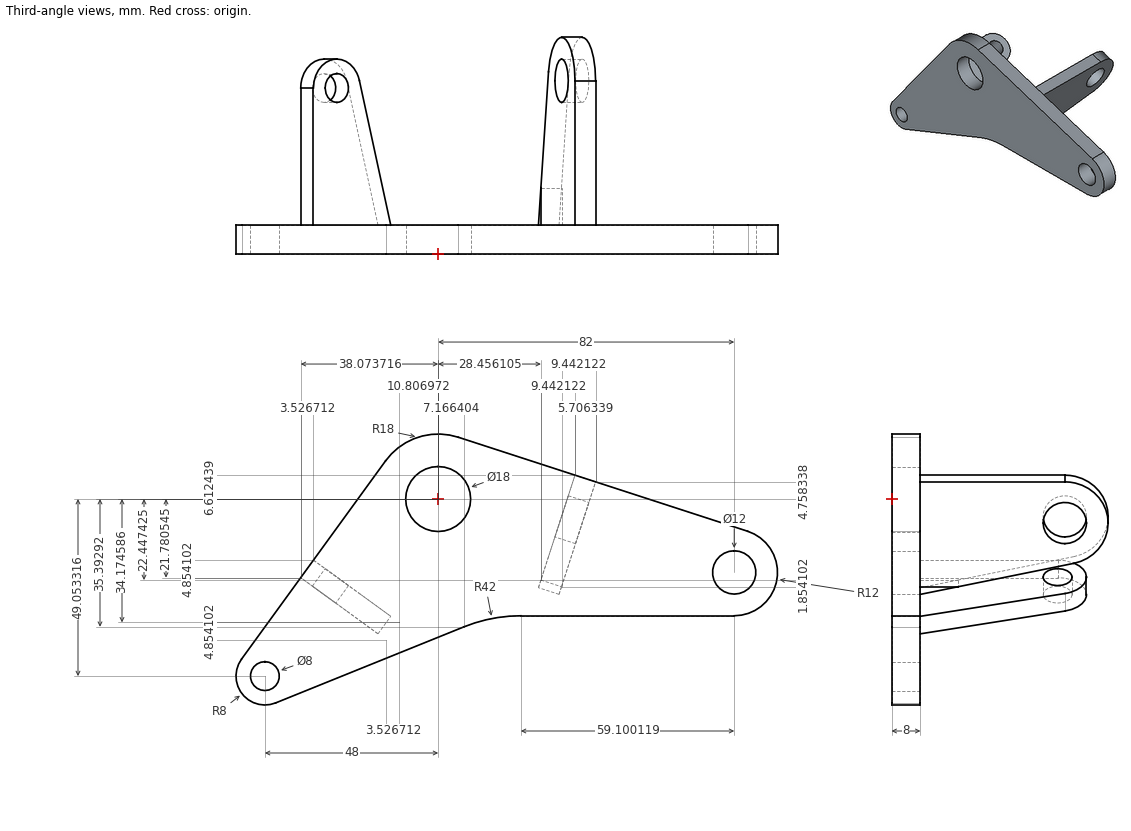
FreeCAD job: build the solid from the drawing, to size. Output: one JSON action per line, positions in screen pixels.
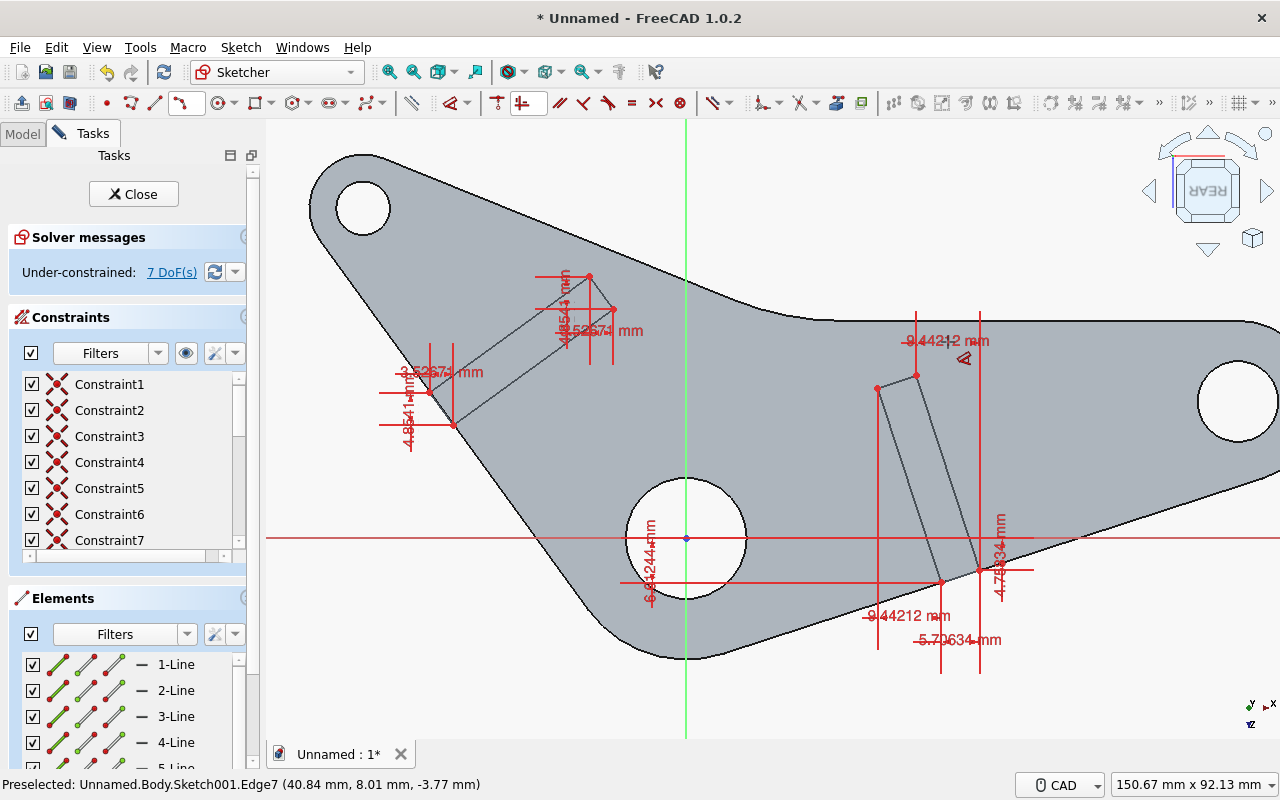
{"action": "scroll", "coordinate": [905, 380], "scroll_direction": "up", "scroll_amount": 6}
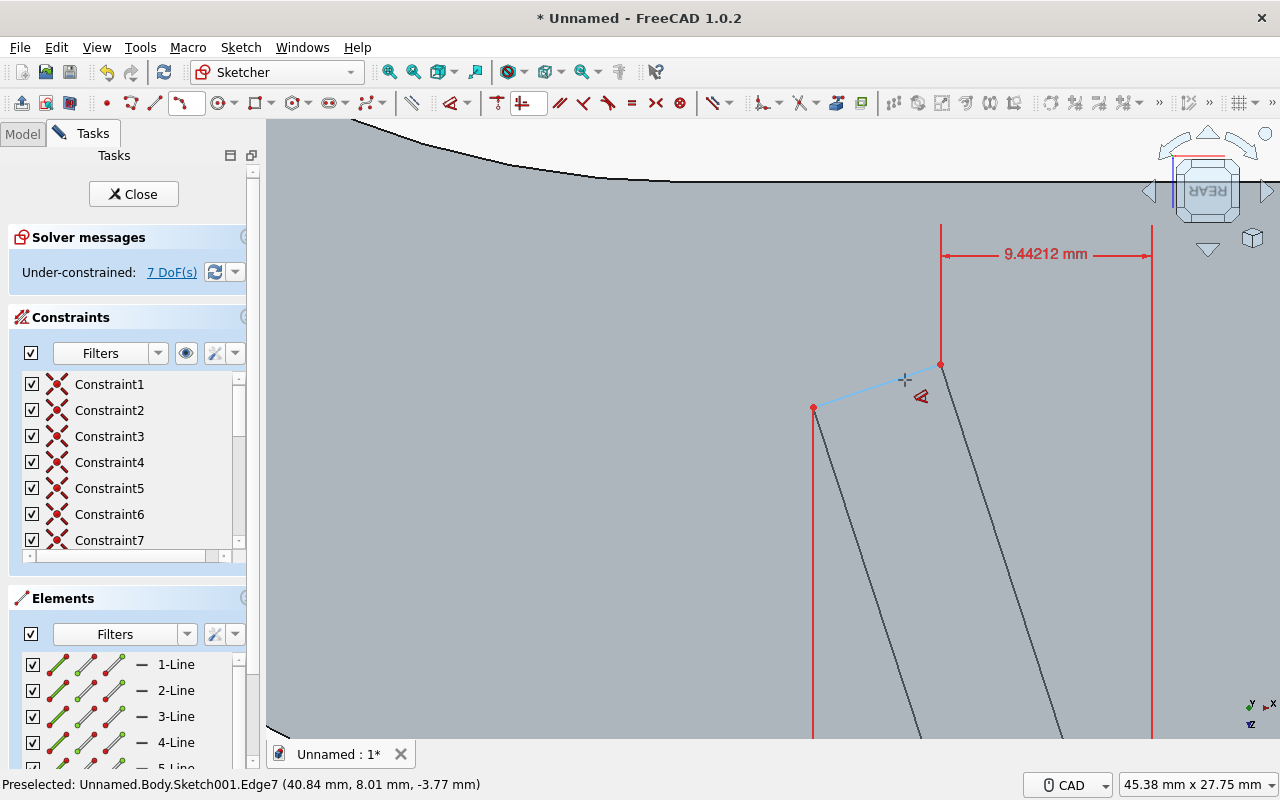
{"action": "left_click", "coordinate": [902, 378]}
{"action": "left_click", "coordinate": [975, 386]}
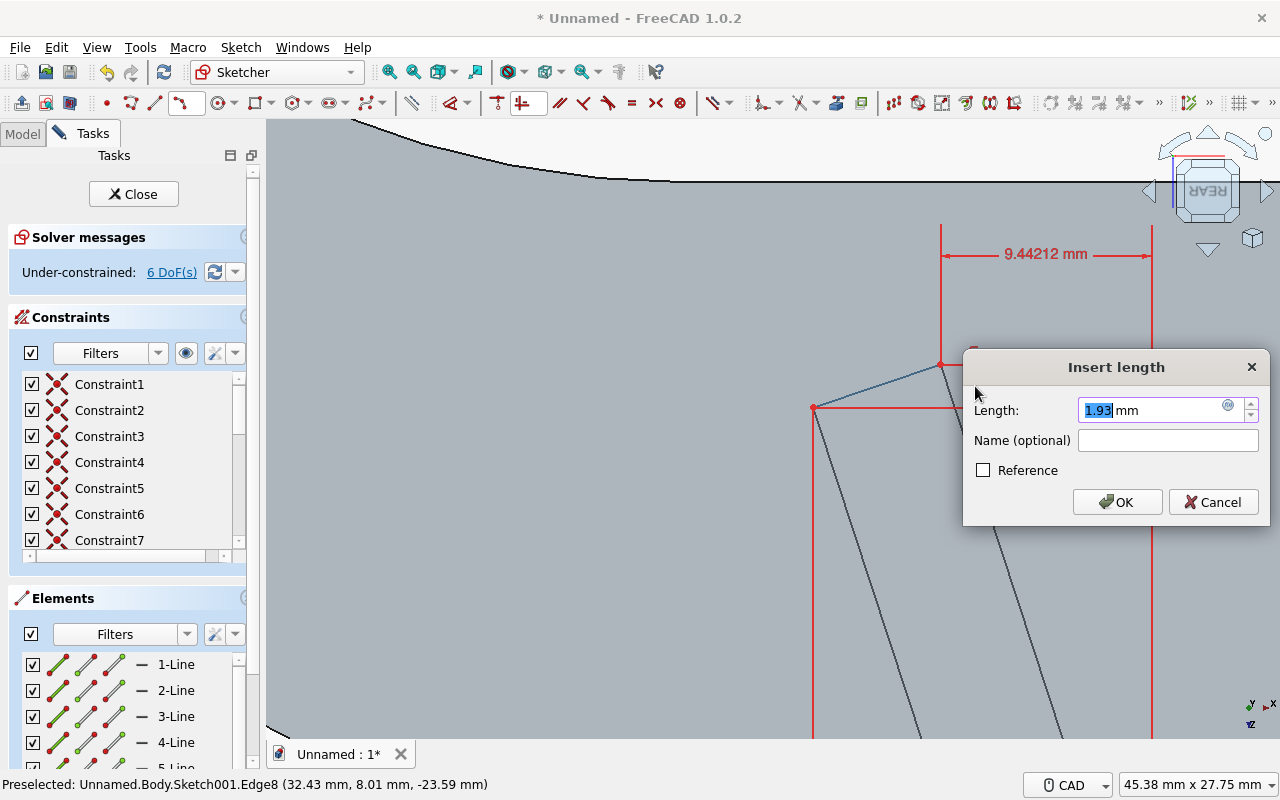
{"action": "type", "text": "1.854102"}
{"action": "key", "text": "Return"}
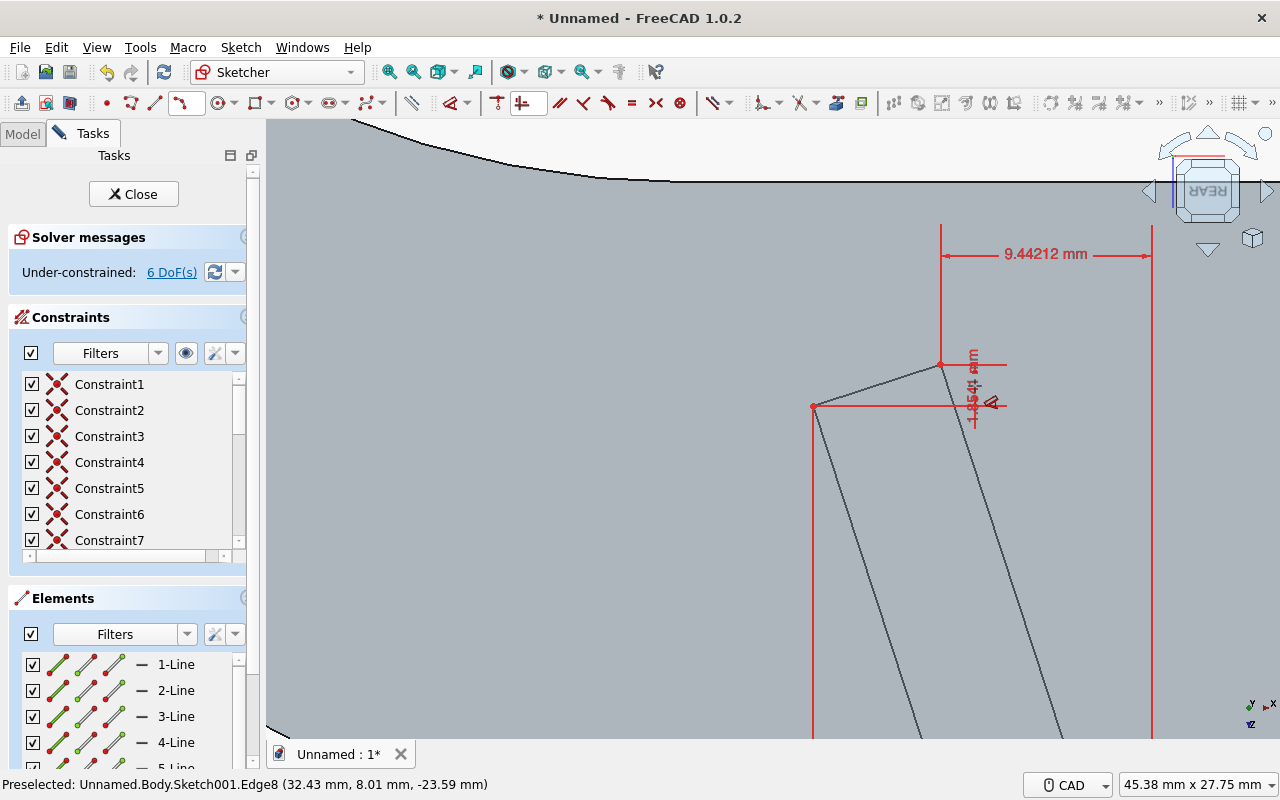
{"action": "scroll", "coordinate": [905, 380], "scroll_direction": "down", "scroll_amount": 6}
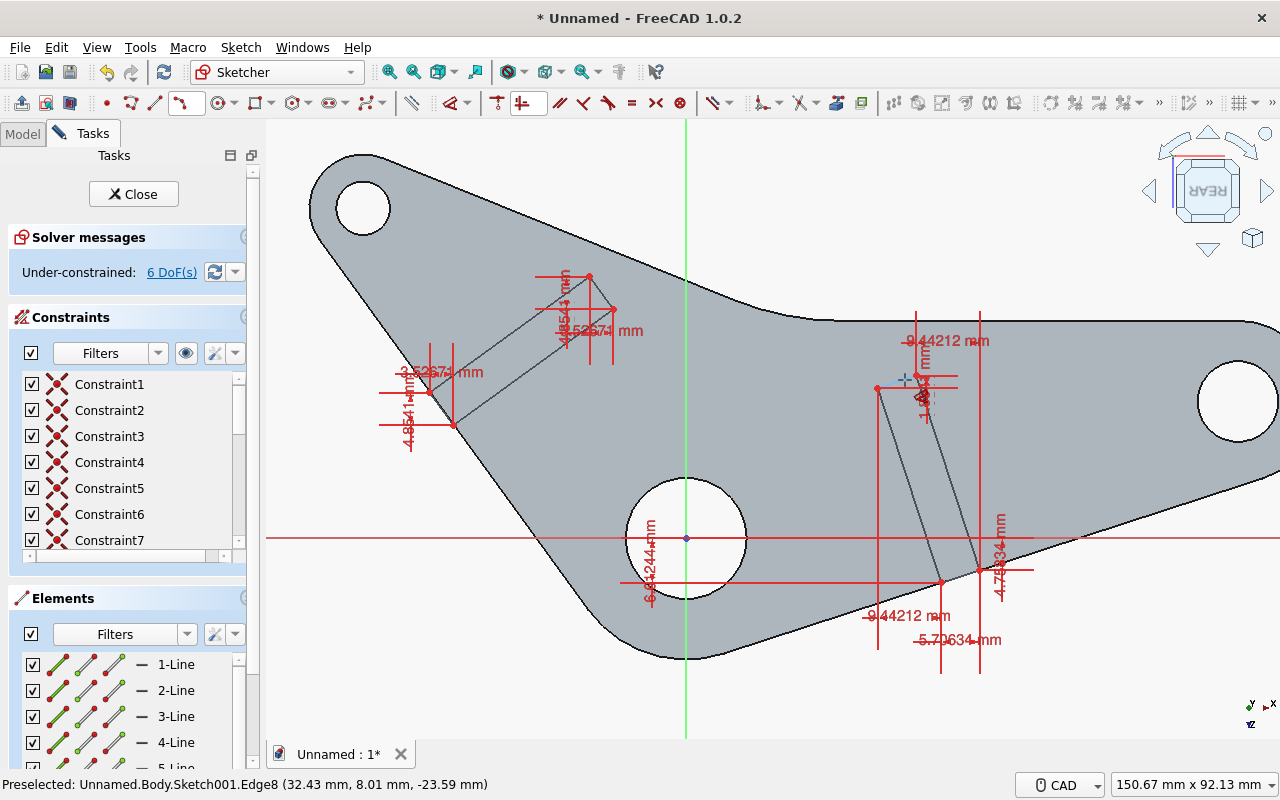
{"action": "left_click", "coordinate": [613, 309]}
{"action": "left_click", "coordinate": [650, 275]}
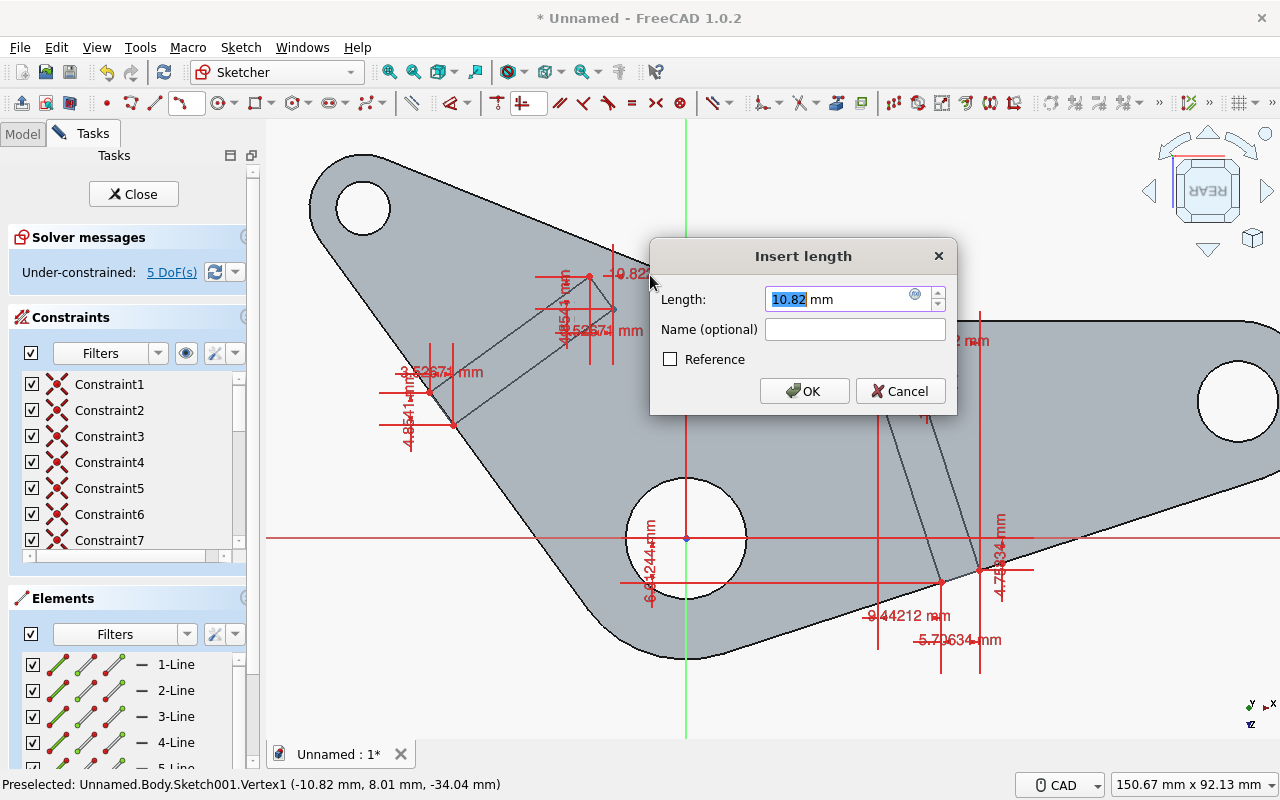
{"action": "type", "text": "10.806972"}
{"action": "key", "text": "Return"}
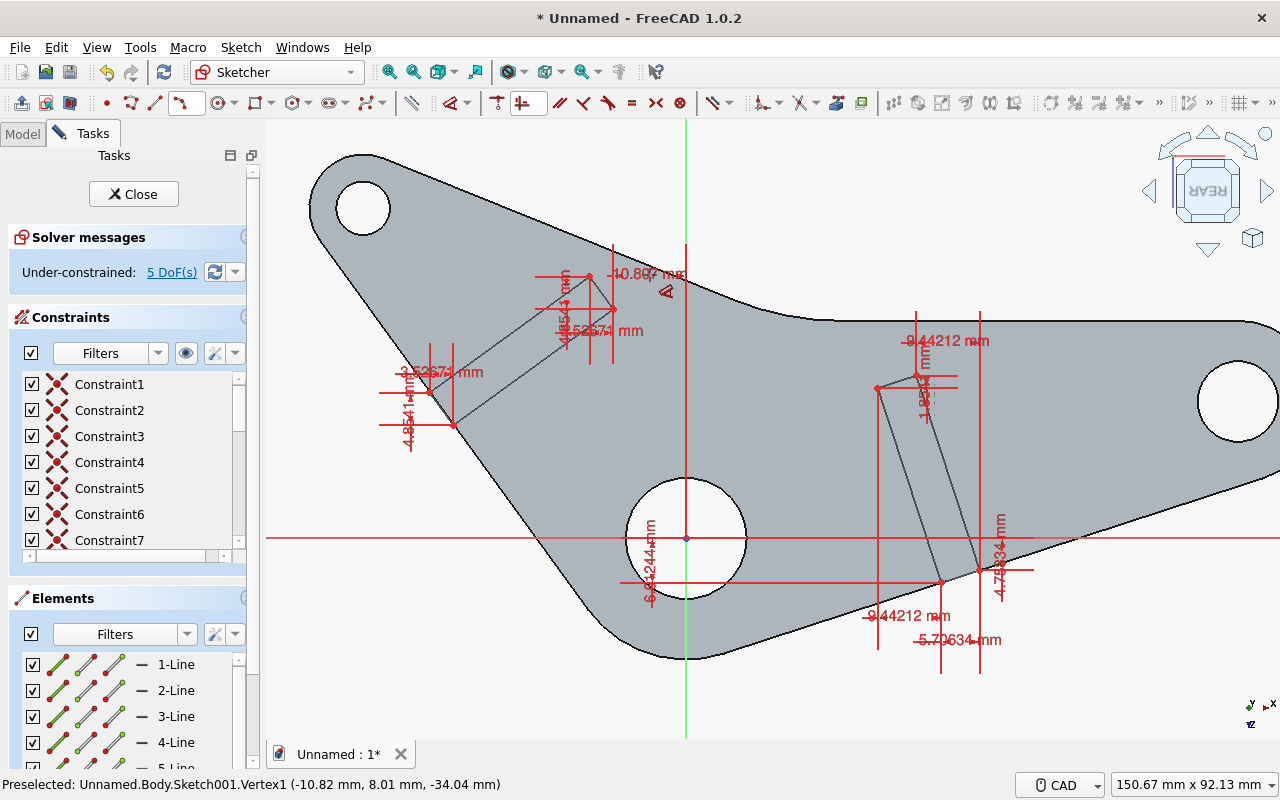
{"action": "left_click", "coordinate": [613, 309]}
{"action": "left_click", "coordinate": [579, 424]}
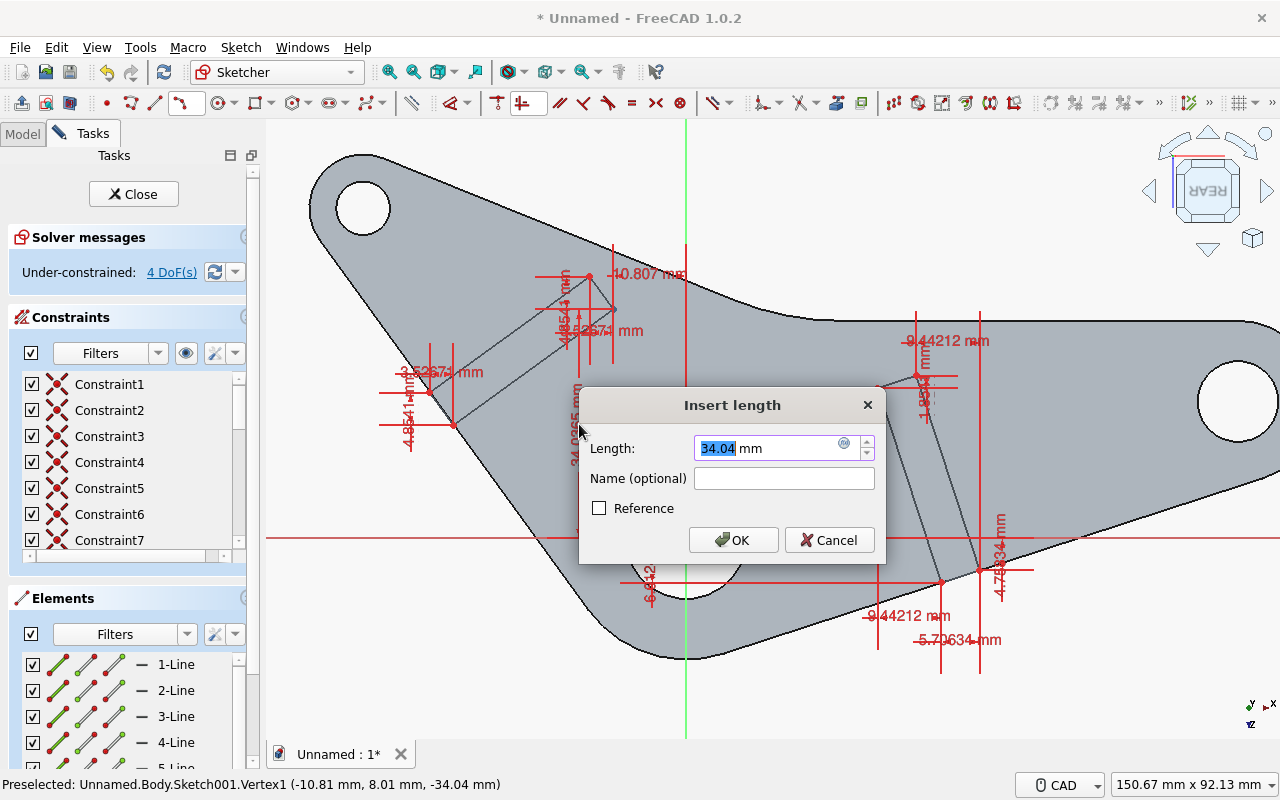
{"action": "type", "text": "34.174586"}
{"action": "key", "text": "Return"}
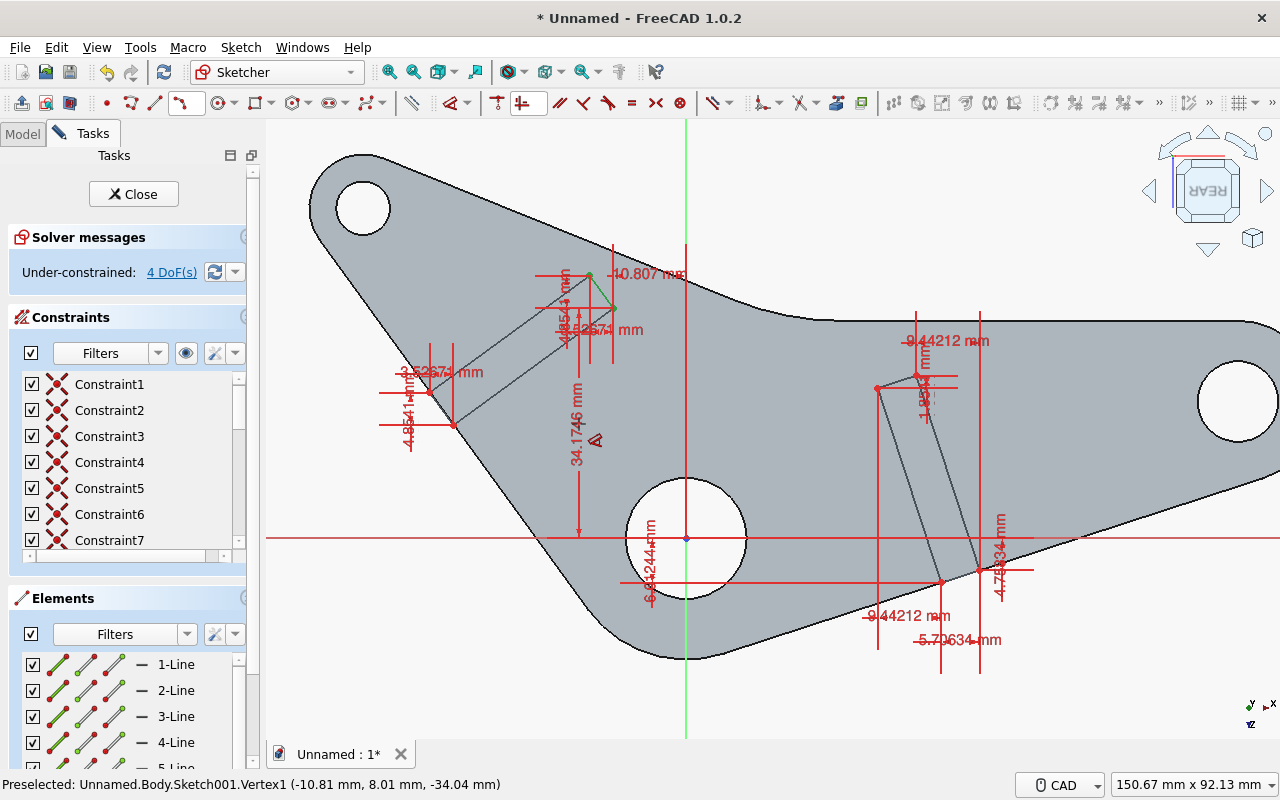
{"action": "left_click", "coordinate": [430, 393]}
{"action": "left_click", "coordinate": [558, 572]}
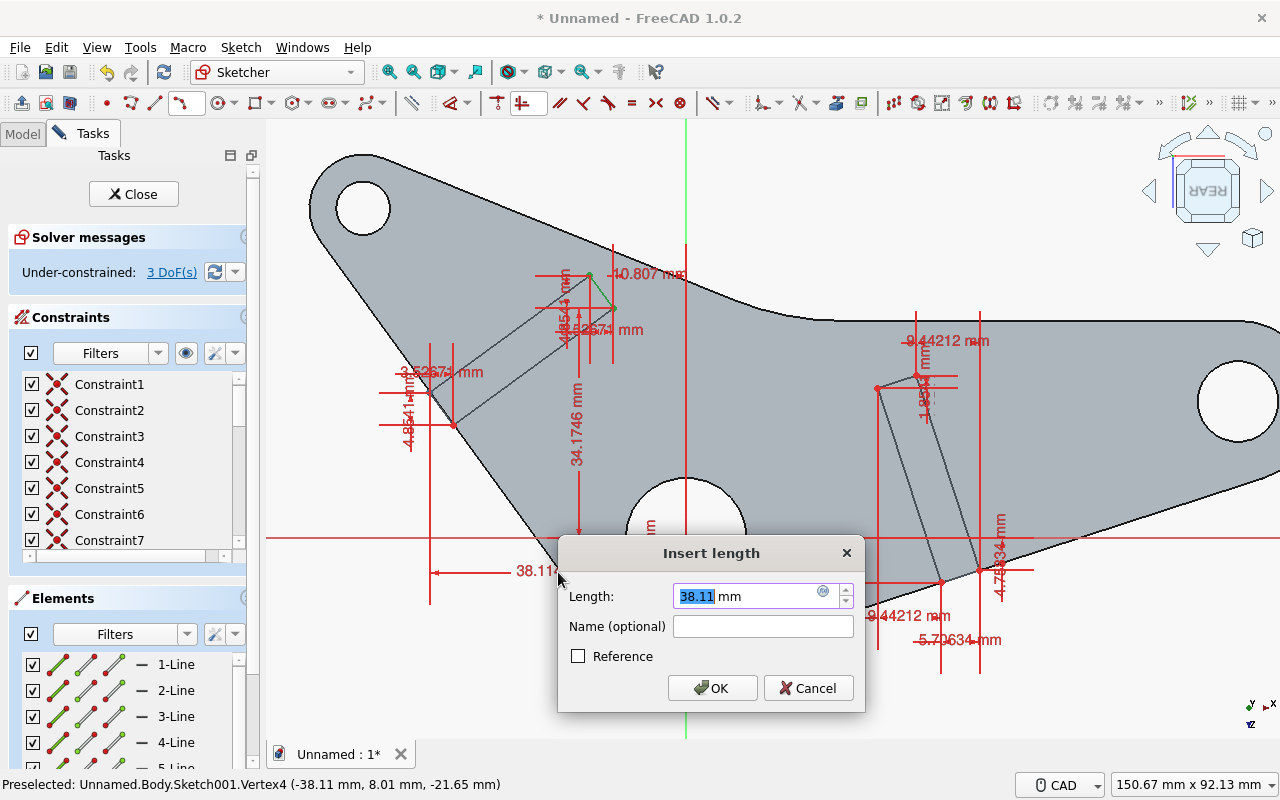
{"action": "type", "text": "38.073716"}
{"action": "key", "text": "Return"}